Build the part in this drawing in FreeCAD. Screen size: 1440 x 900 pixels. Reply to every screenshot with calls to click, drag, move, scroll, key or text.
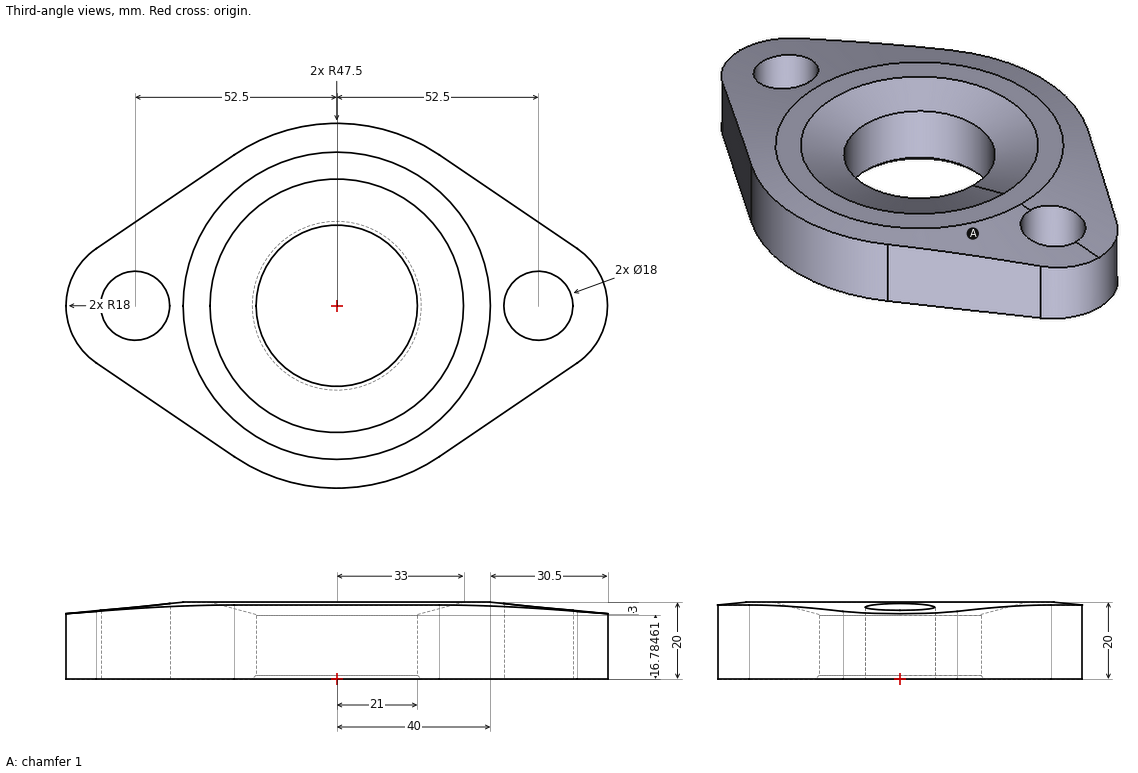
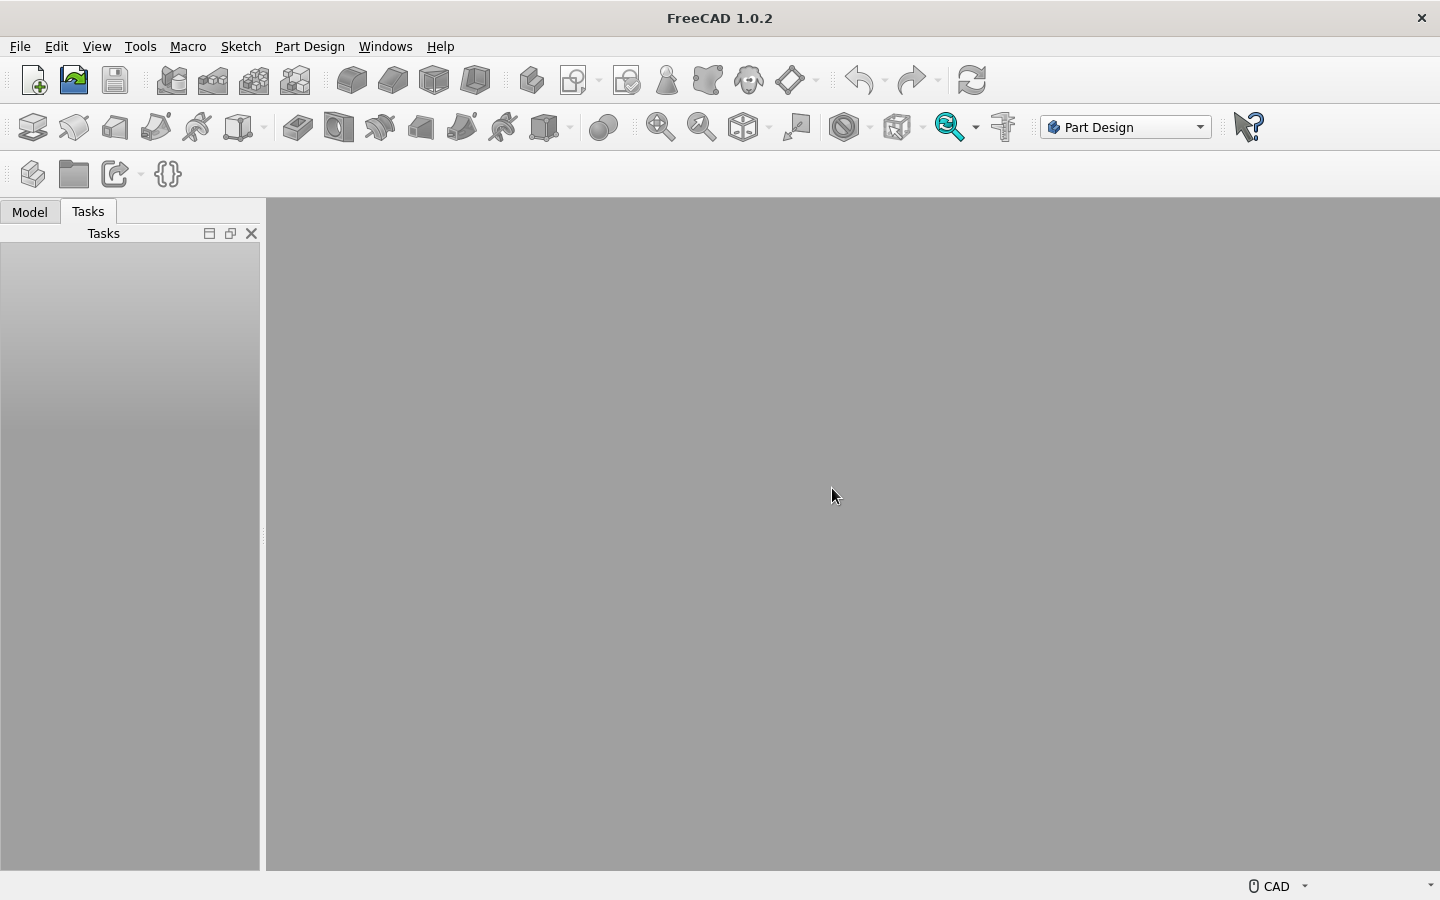
key(ctrl+n)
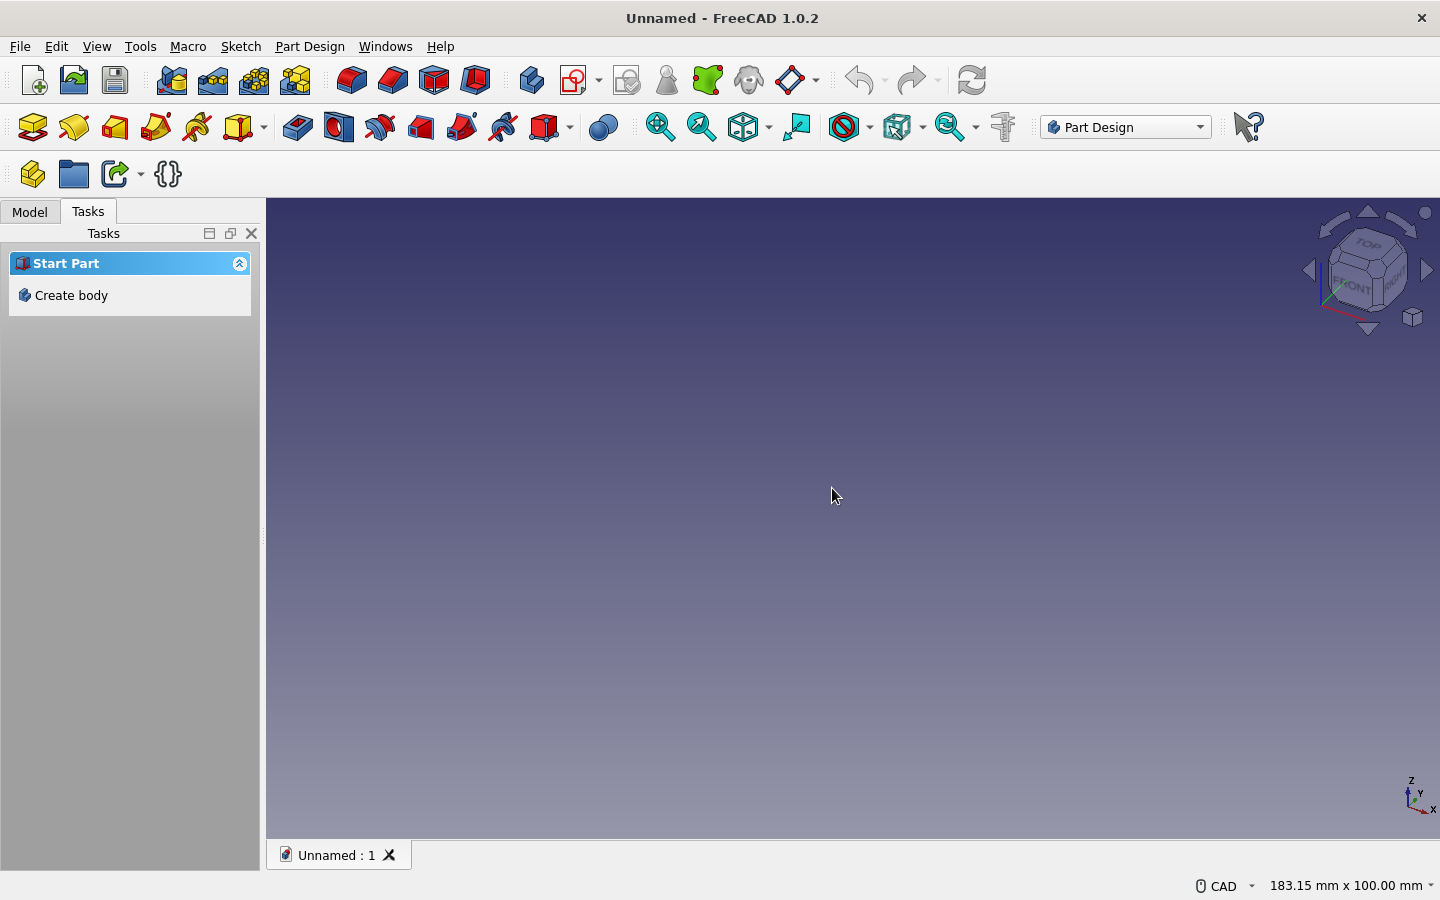
click(572, 80)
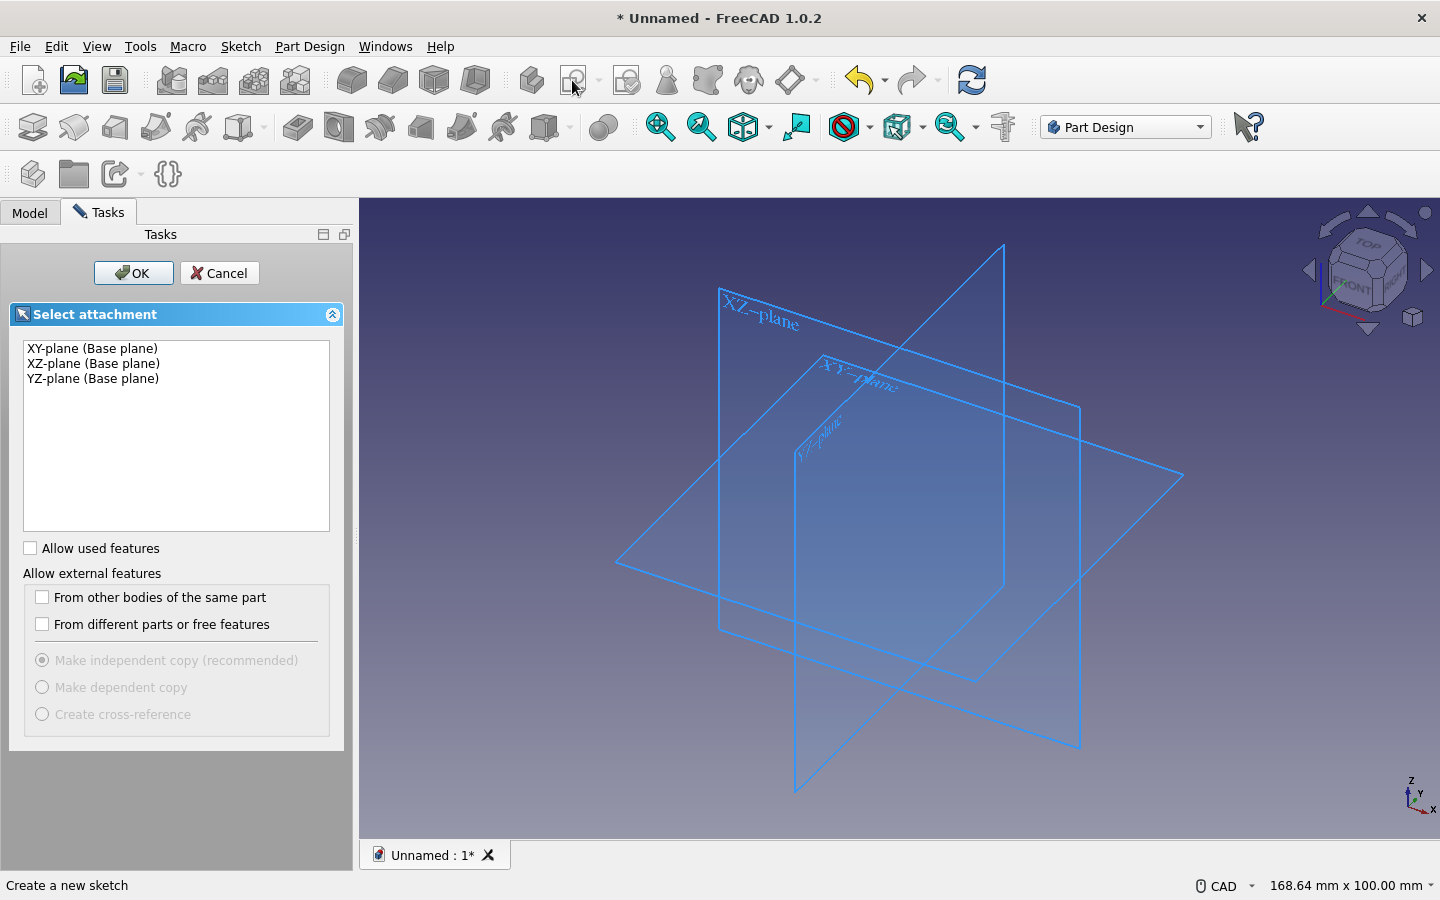
click(84, 348)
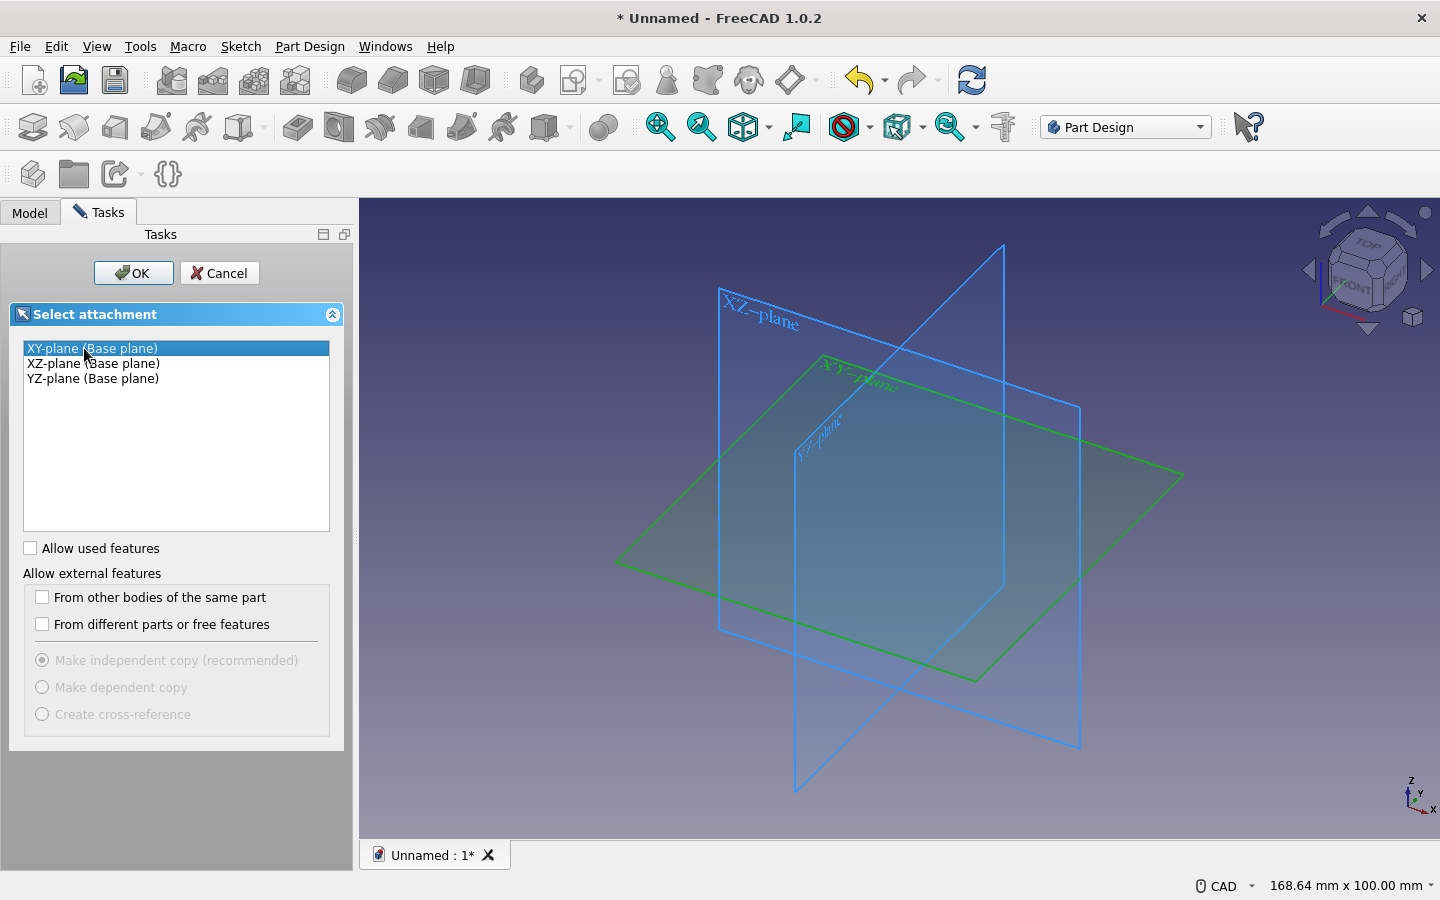
click(134, 273)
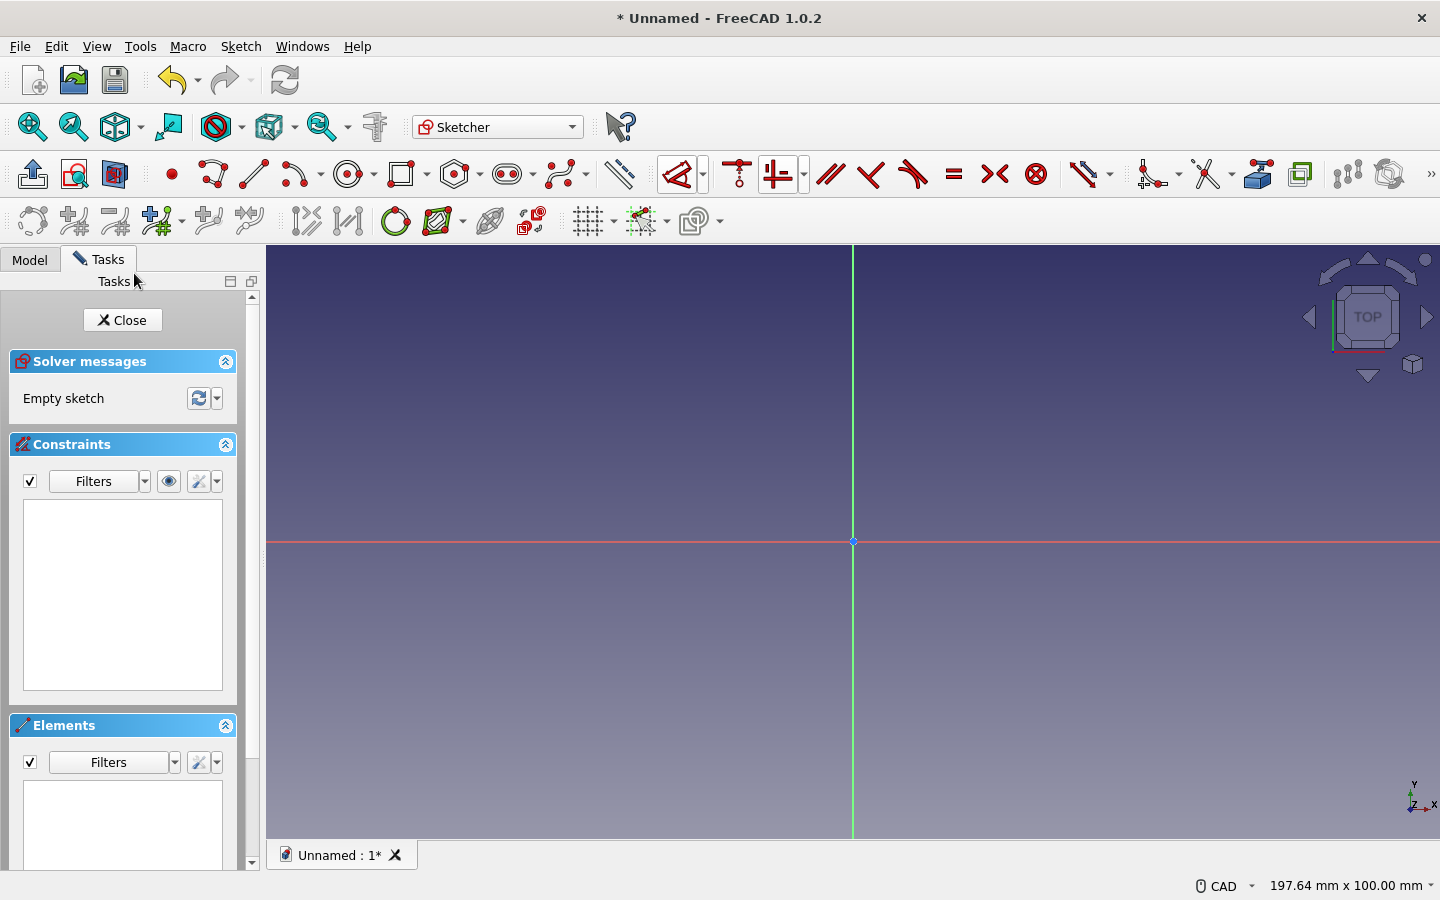
scroll(645, 542, down, 2)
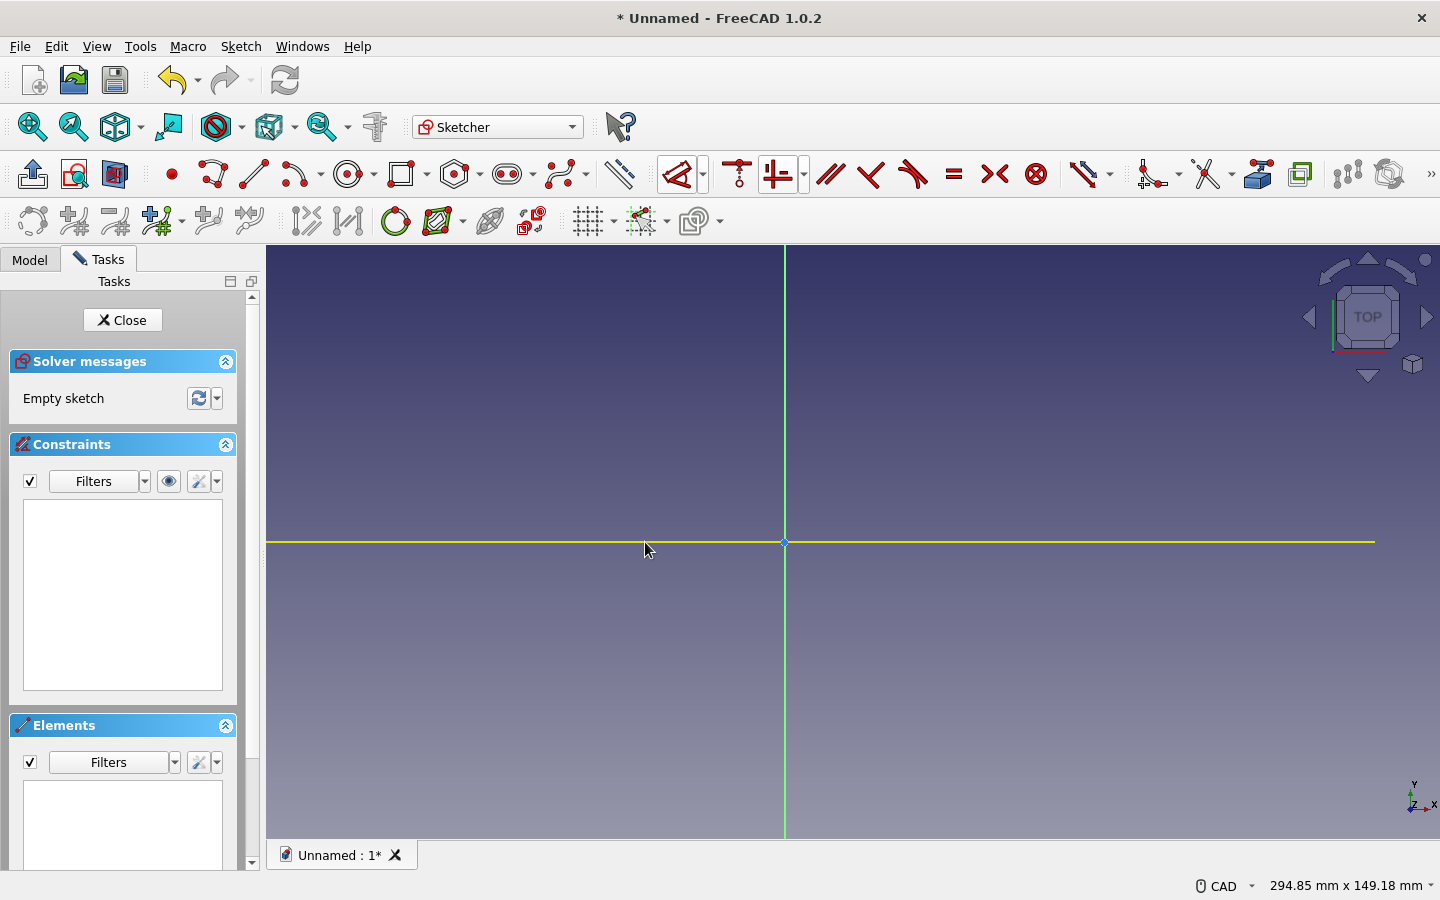
key(g)
key(l)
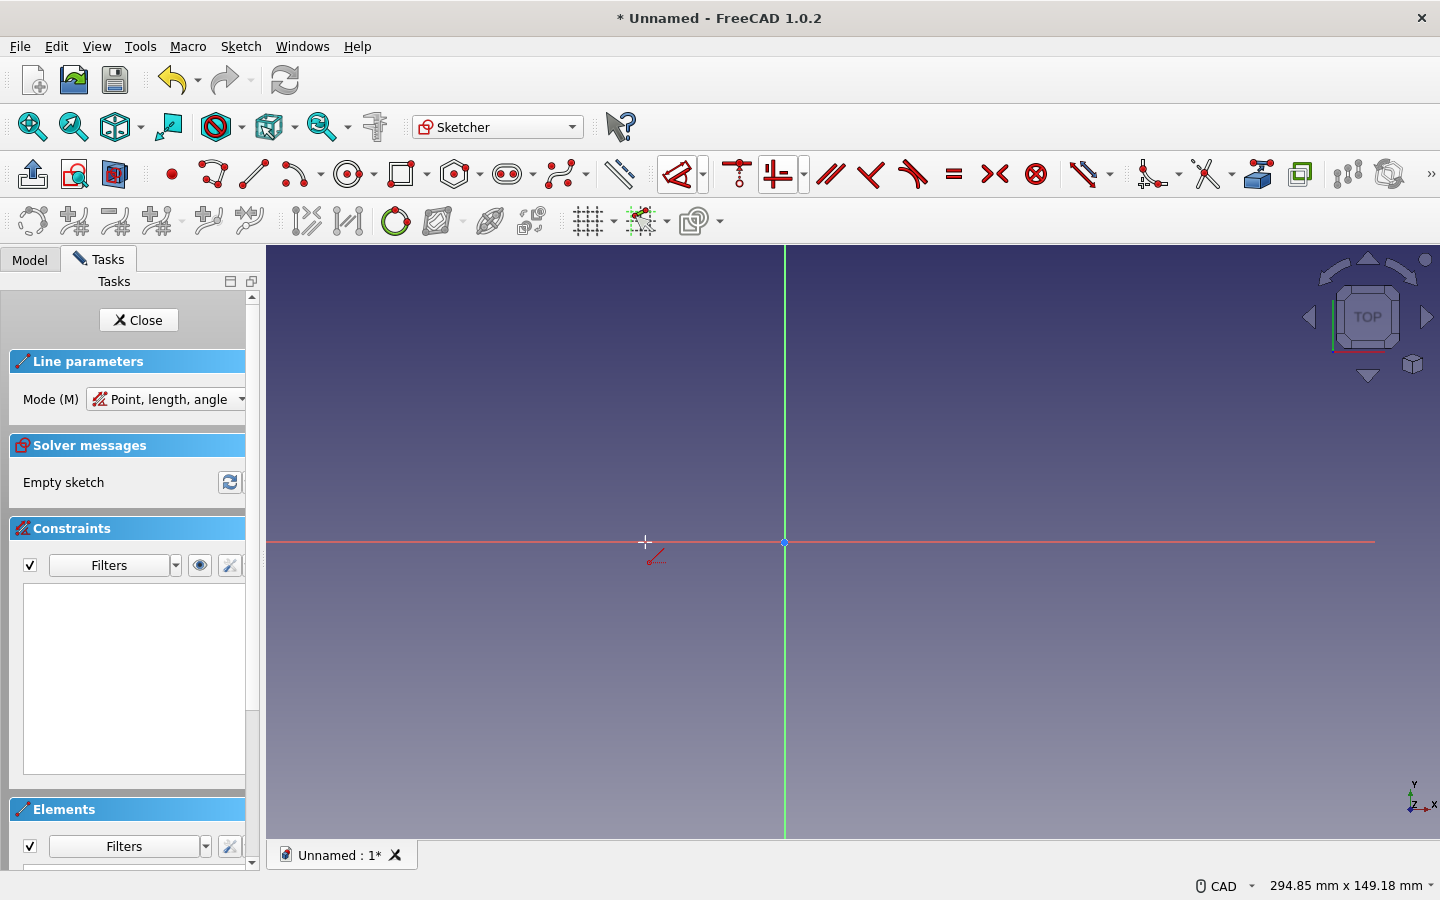
click(1034, 483)
click(891, 386)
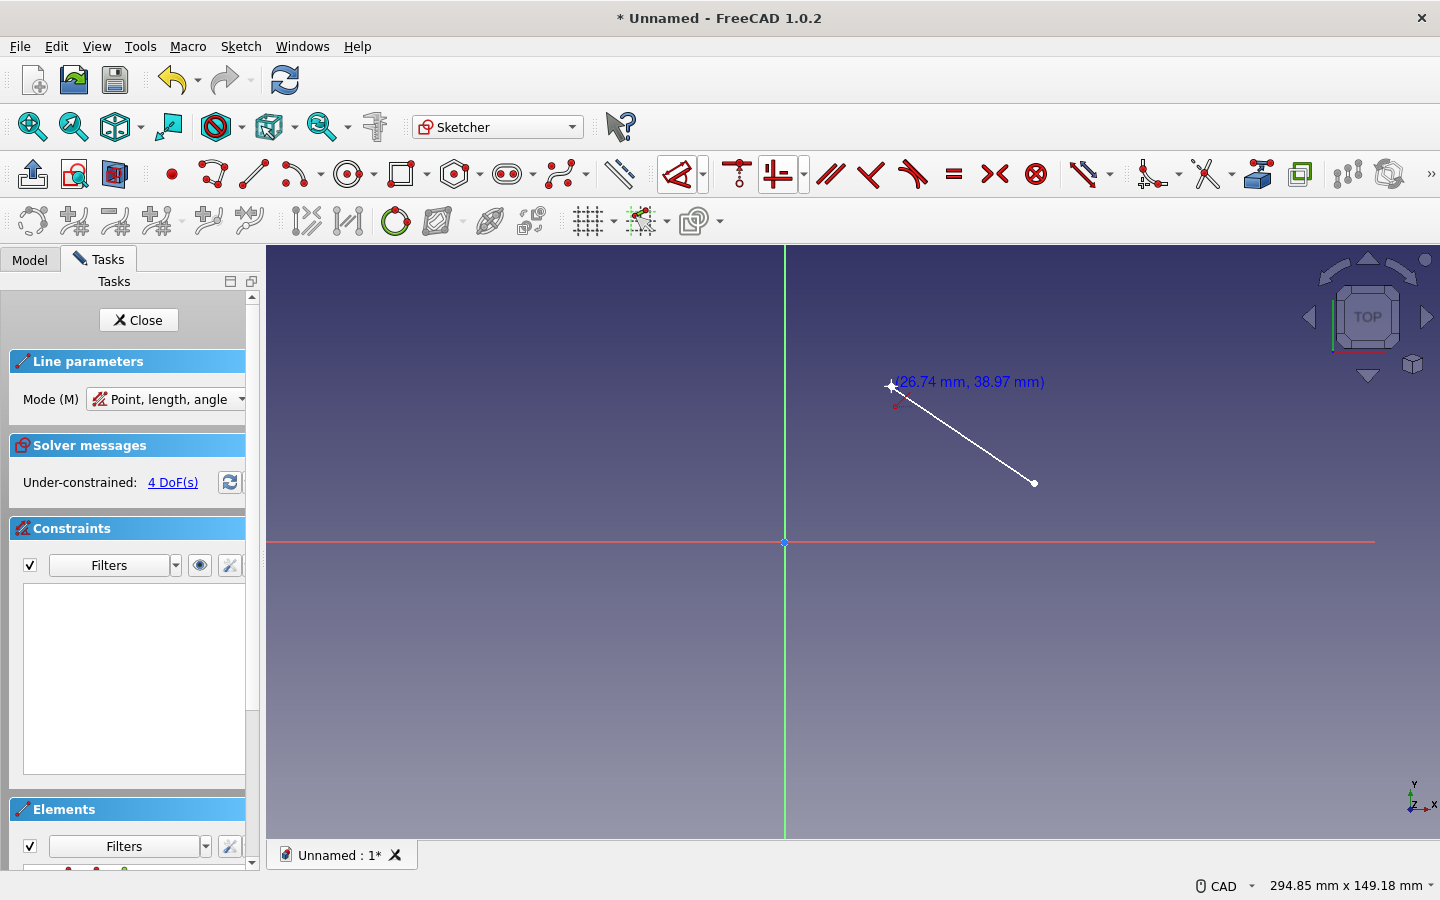
click(678, 386)
click(535, 483)